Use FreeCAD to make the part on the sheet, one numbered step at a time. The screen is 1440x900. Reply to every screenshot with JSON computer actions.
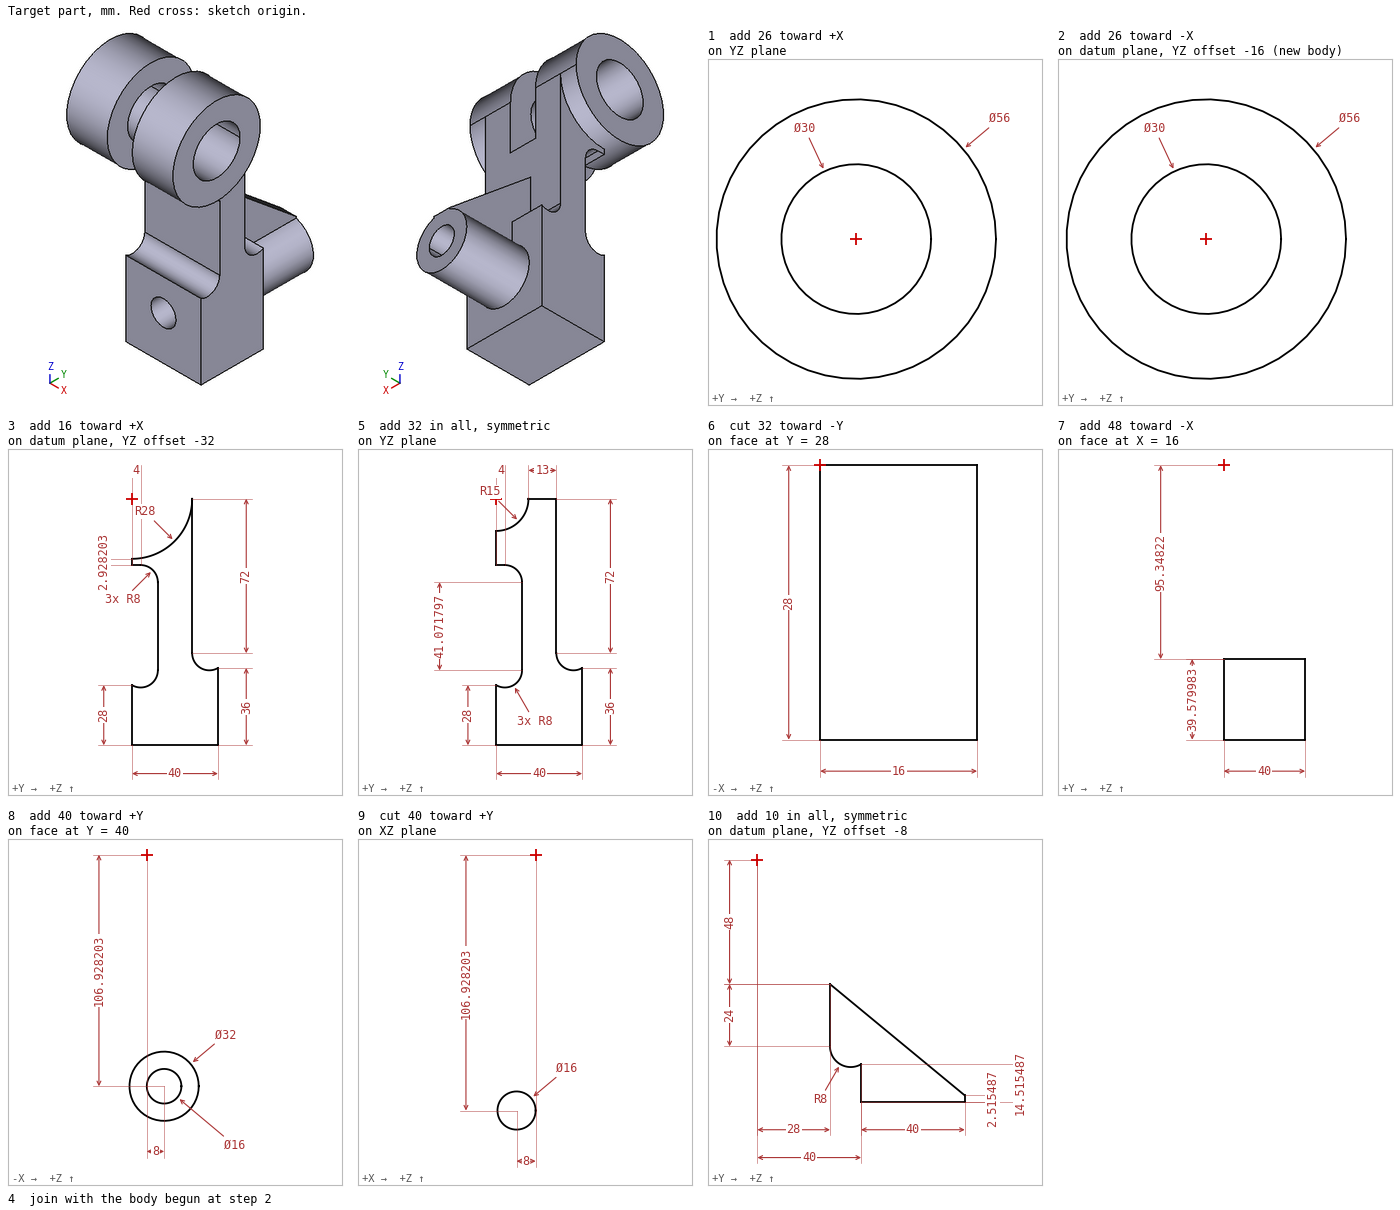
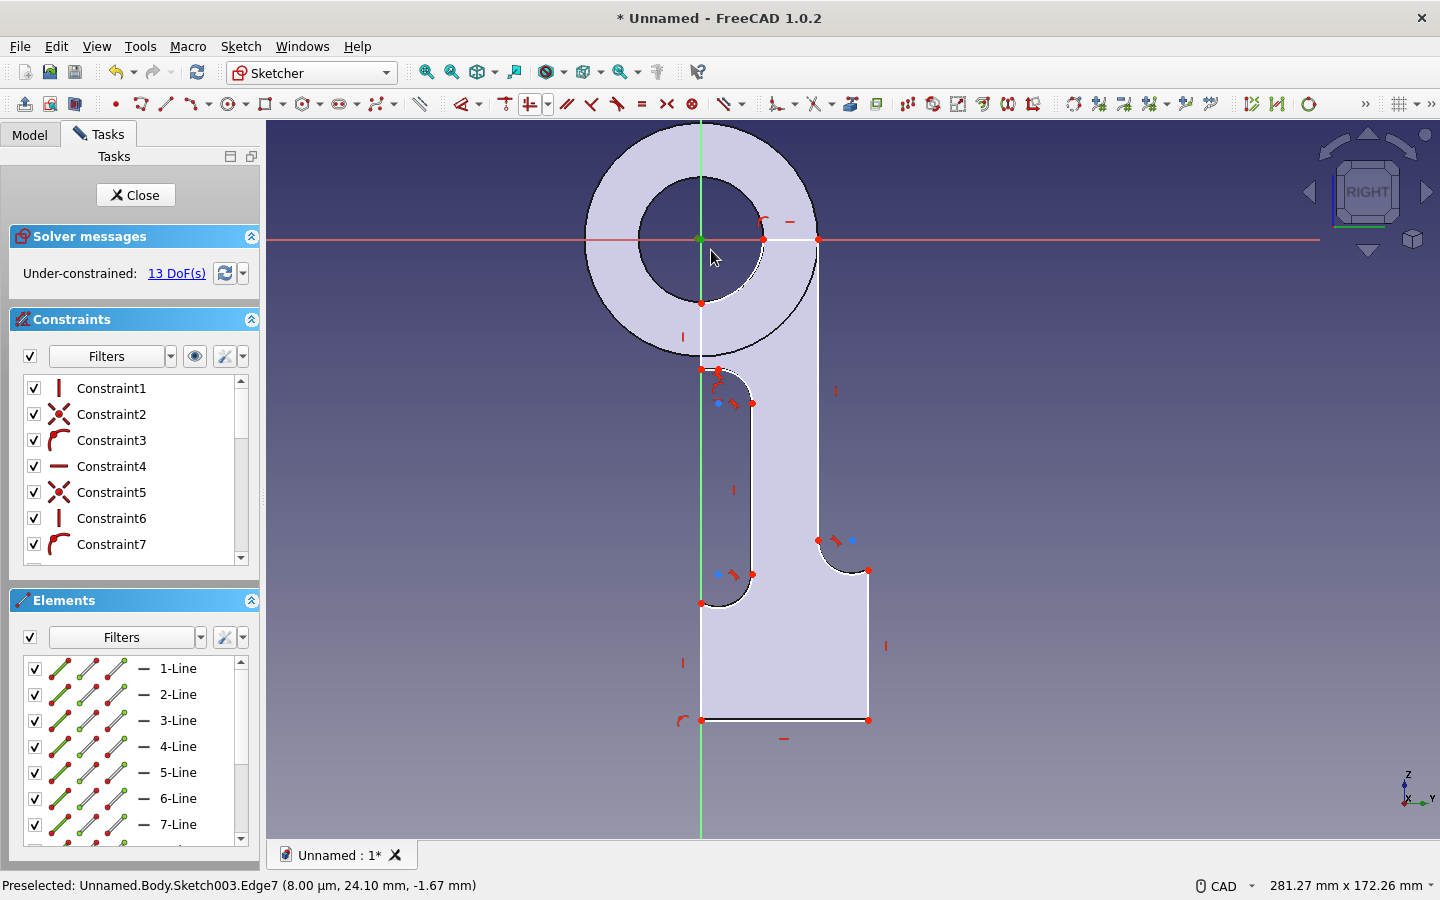
{"action": "left_click", "coordinate": [505, 104]}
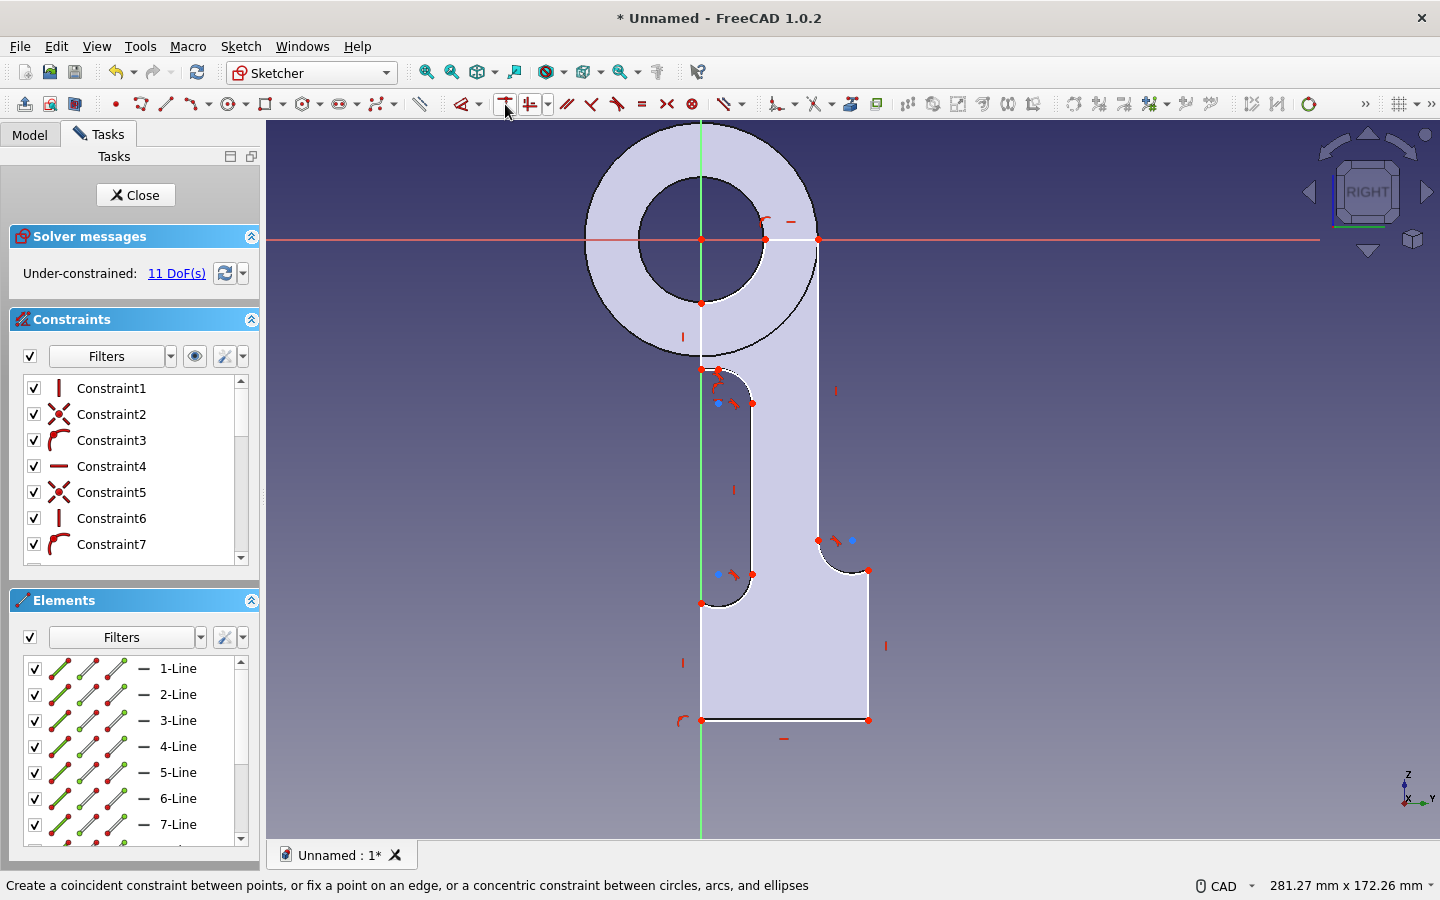
{"action": "left_click", "coordinate": [722, 608]}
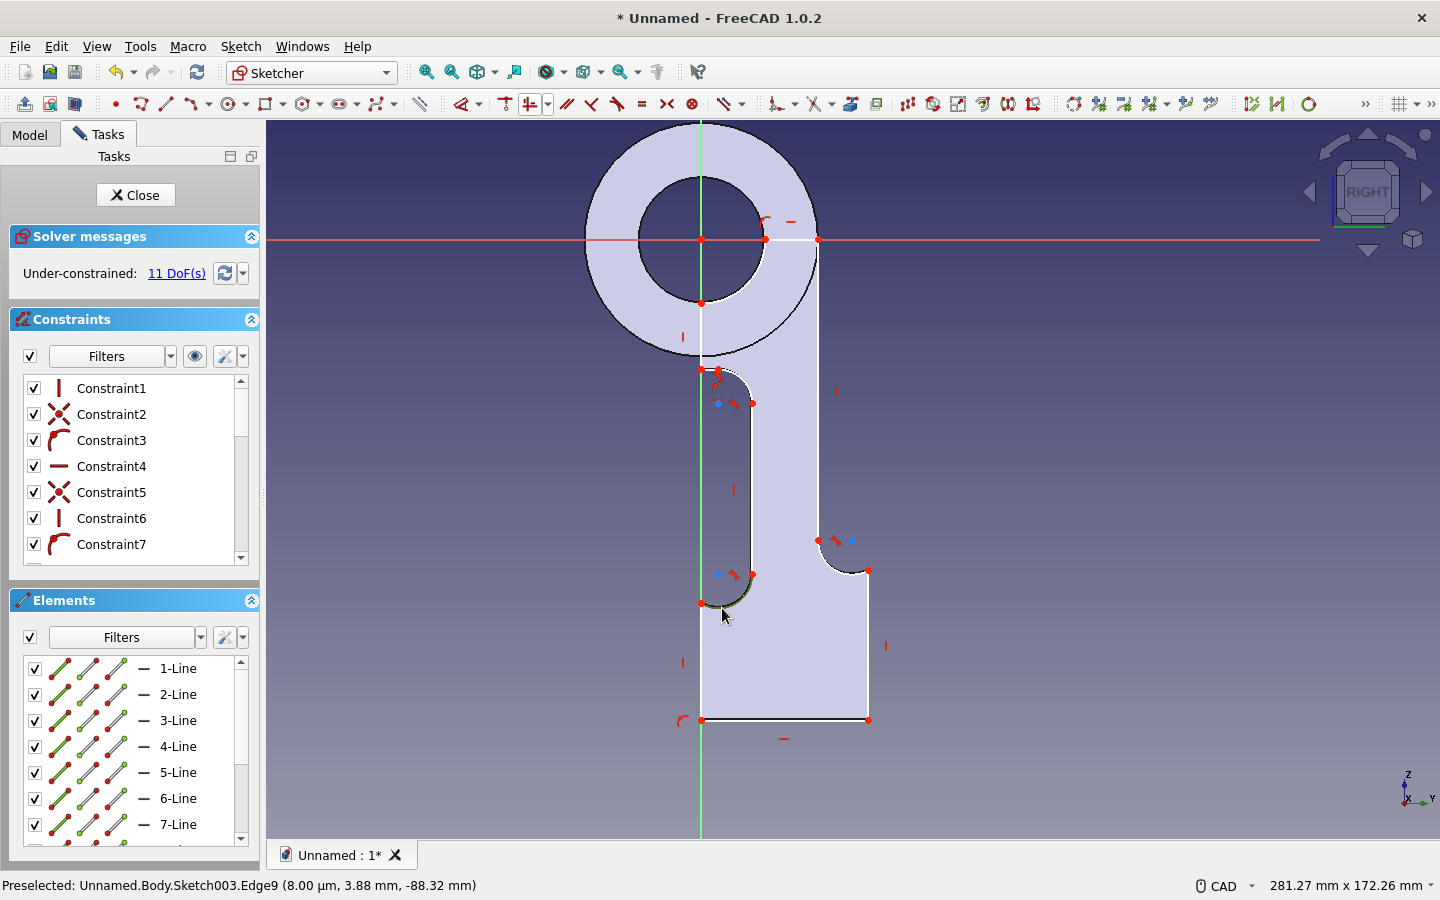
{"action": "left_click", "coordinate": [748, 388]}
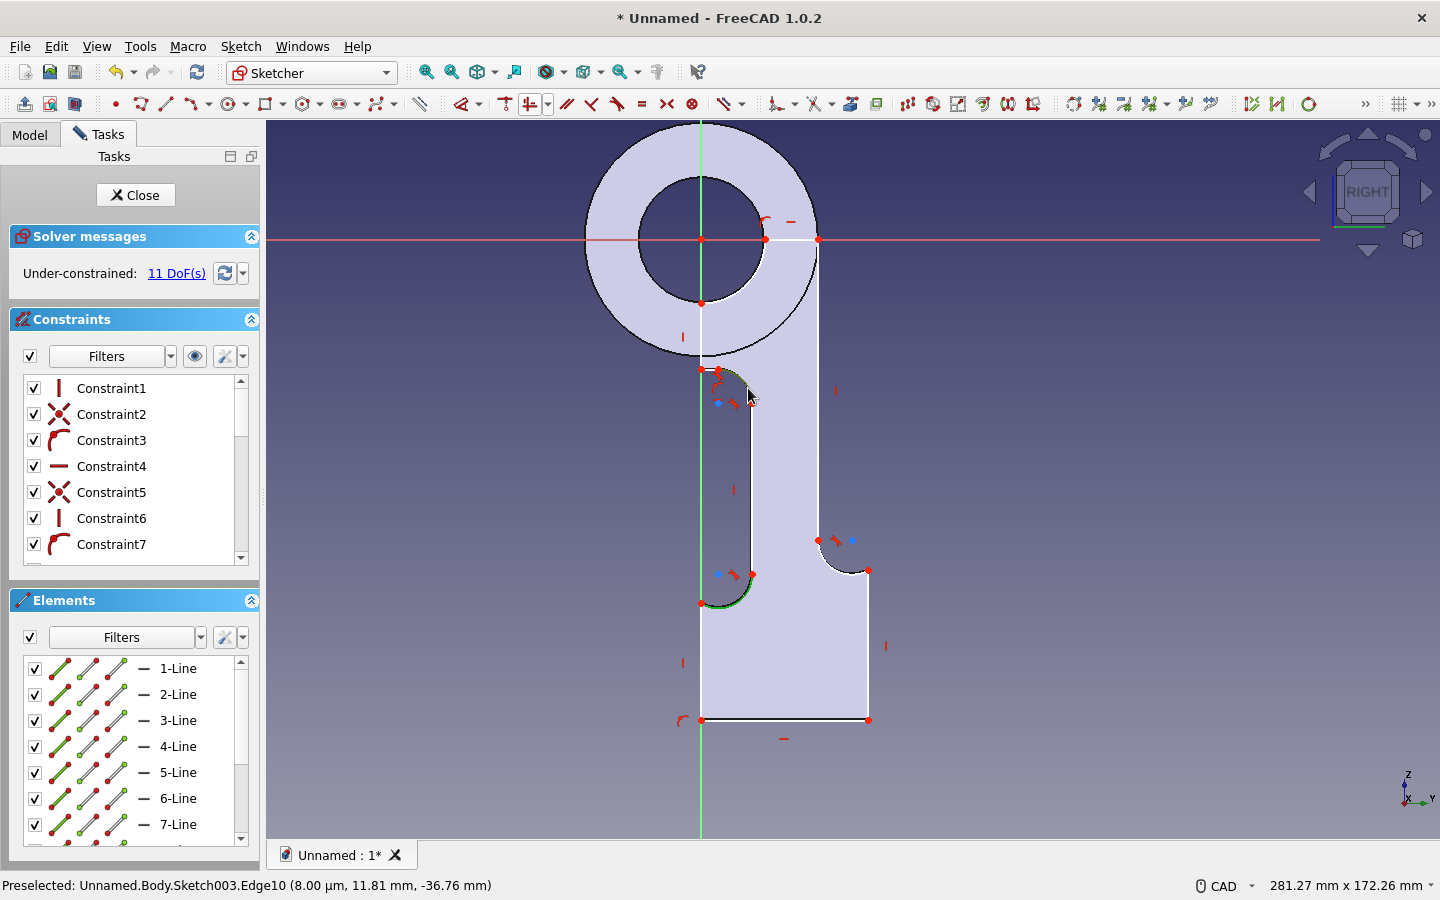
{"action": "left_click", "coordinate": [825, 560]}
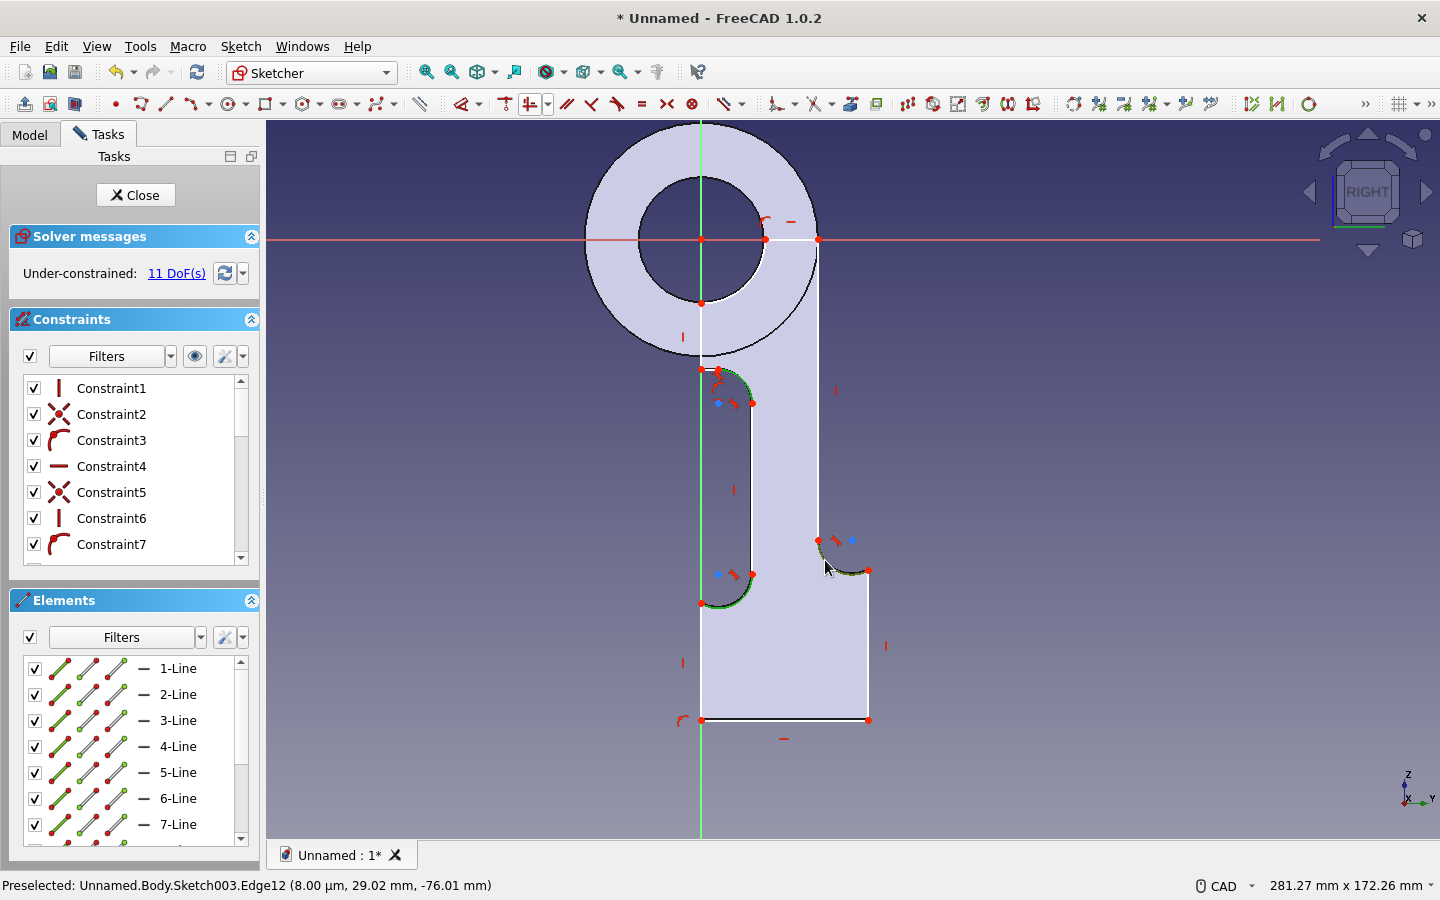
{"action": "key", "text": "e"}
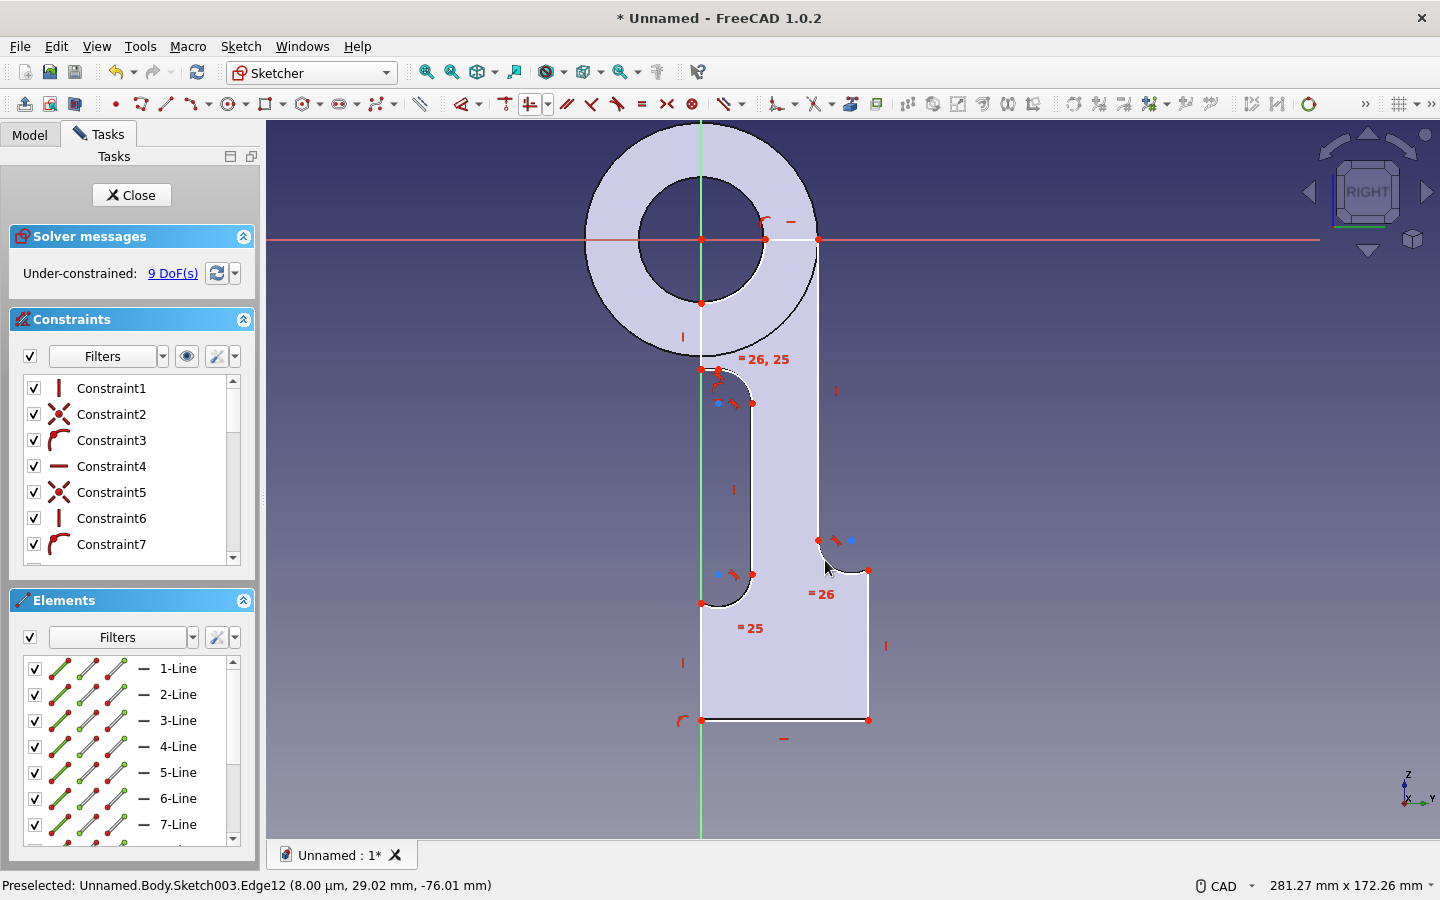
{"action": "key", "text": "d"}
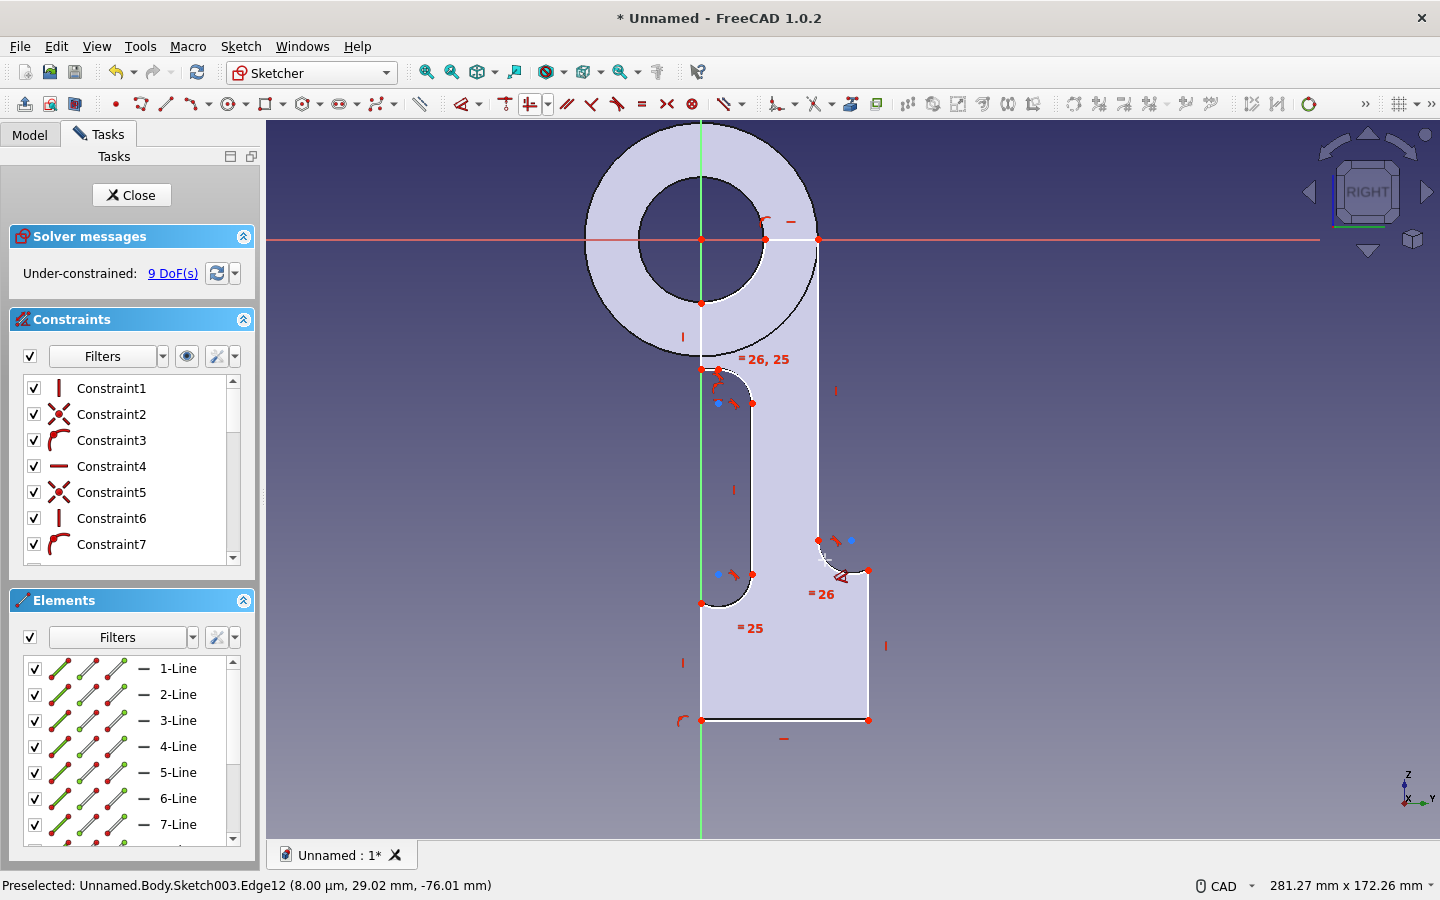
{"action": "left_click", "coordinate": [722, 608]}
{"action": "left_click", "coordinate": [725, 640]}